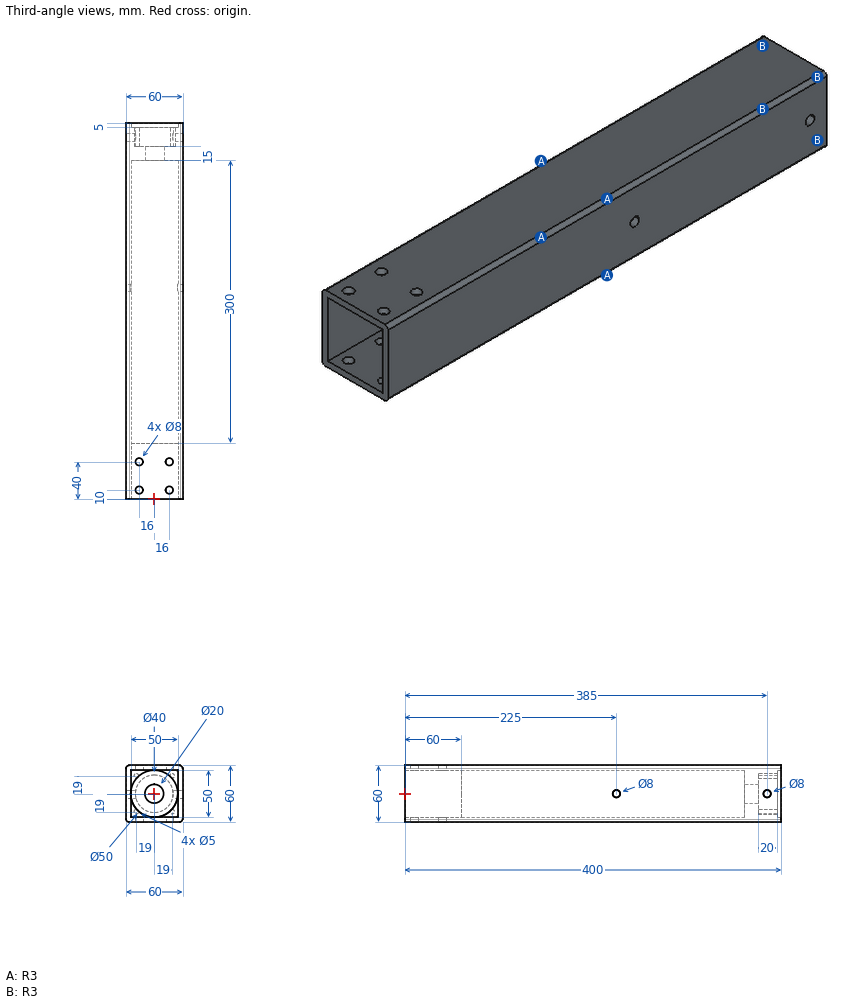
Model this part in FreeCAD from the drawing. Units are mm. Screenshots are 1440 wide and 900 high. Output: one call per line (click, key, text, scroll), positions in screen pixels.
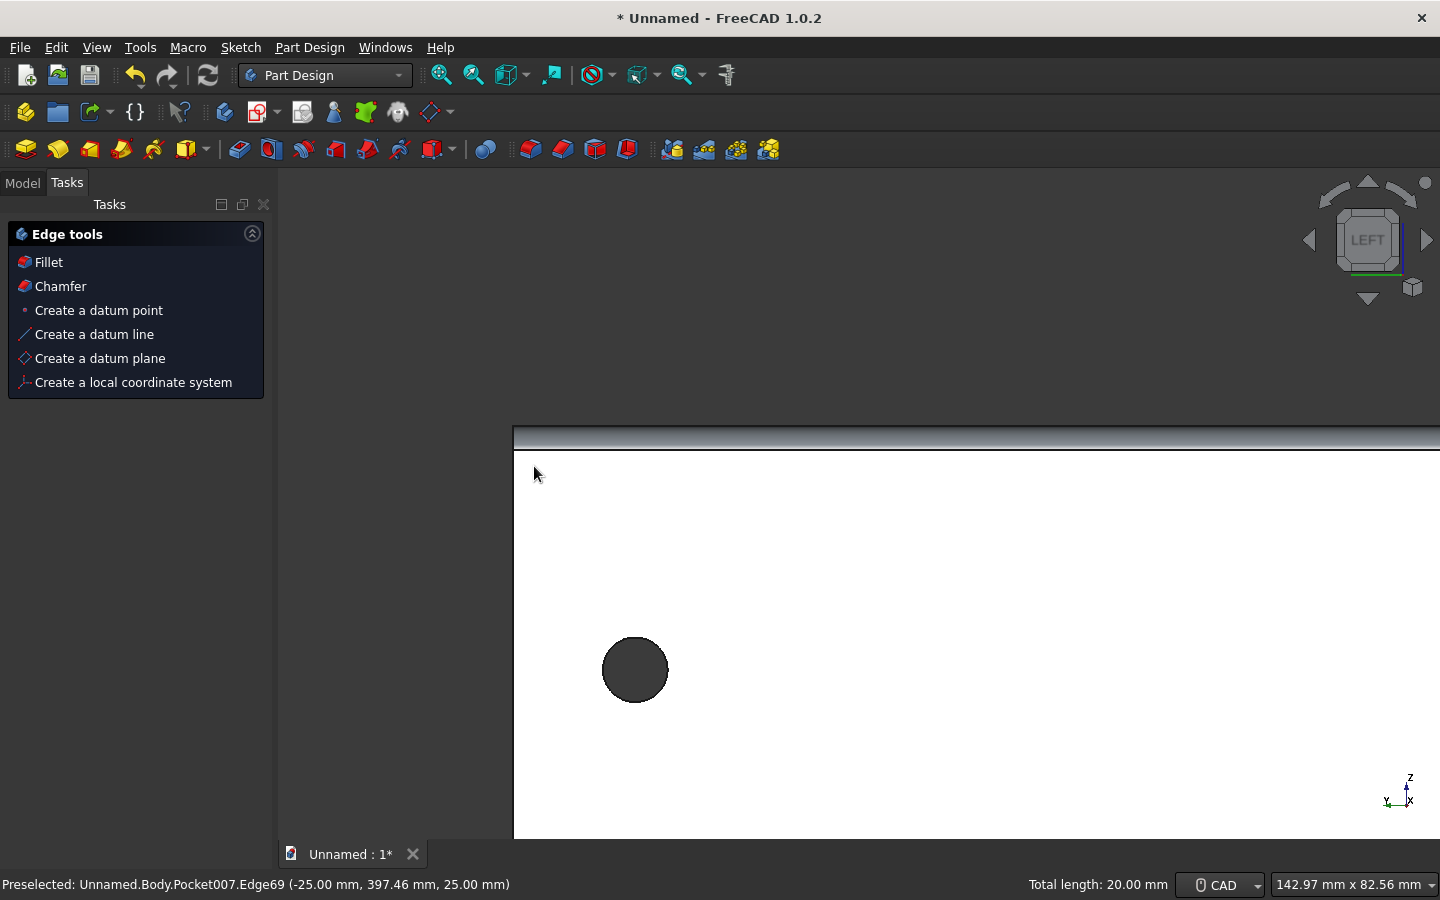
click(532, 150)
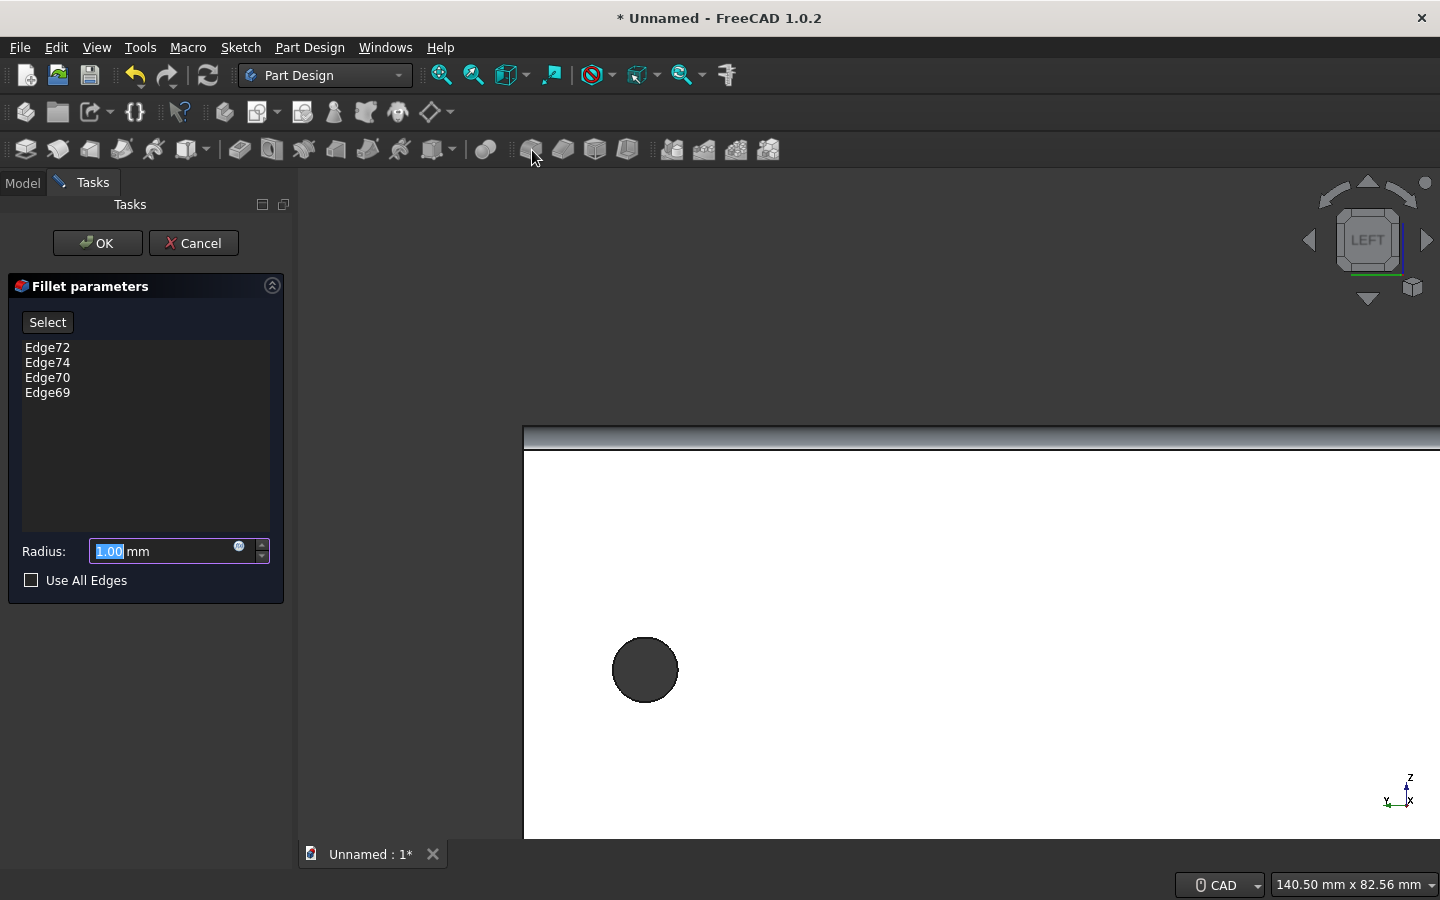
text(3)
key(Tab)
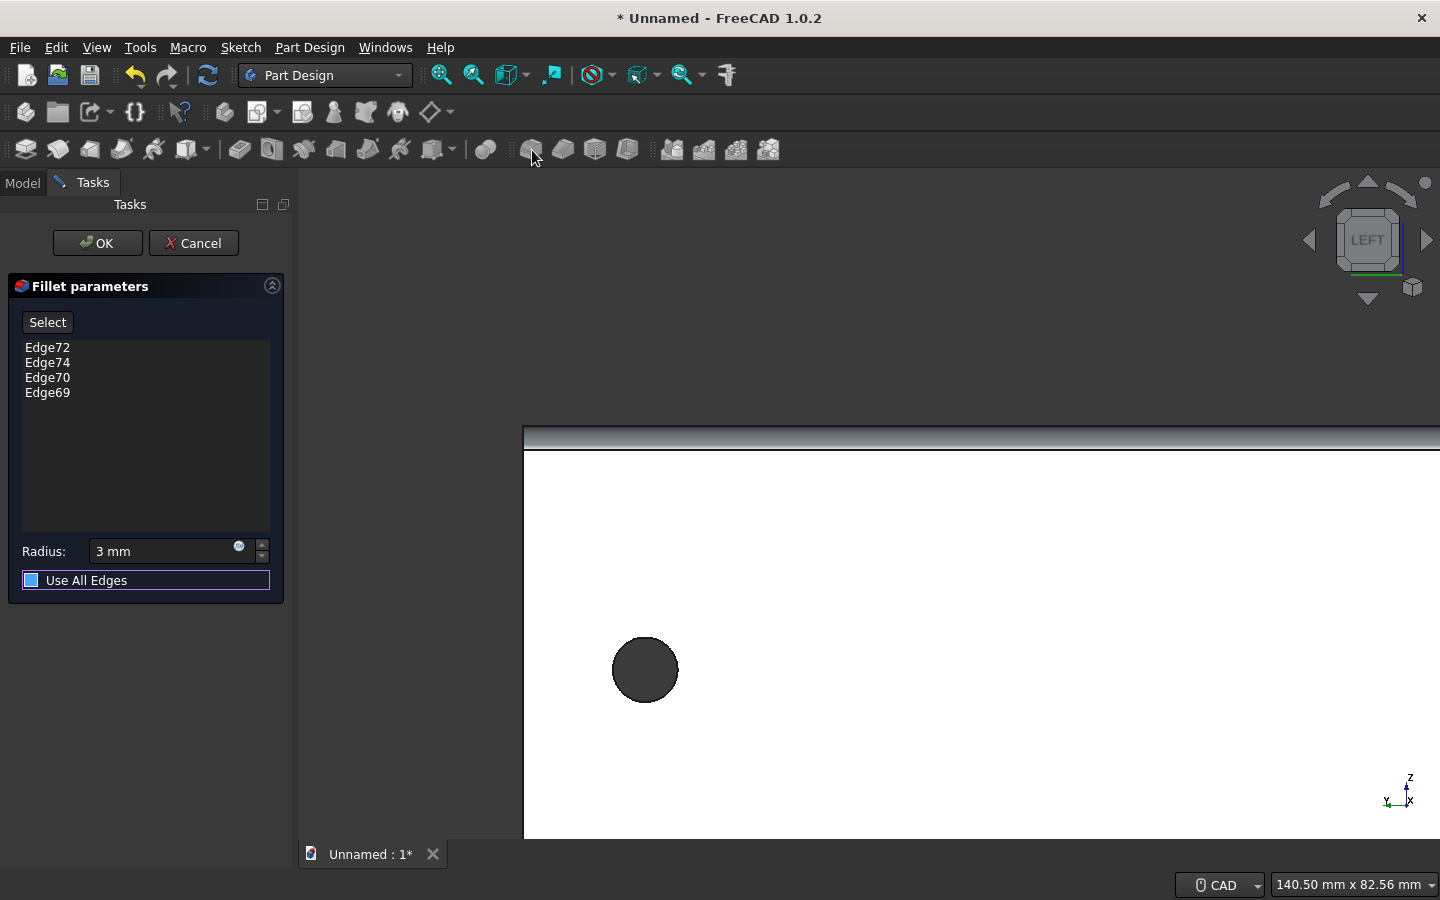
click(98, 243)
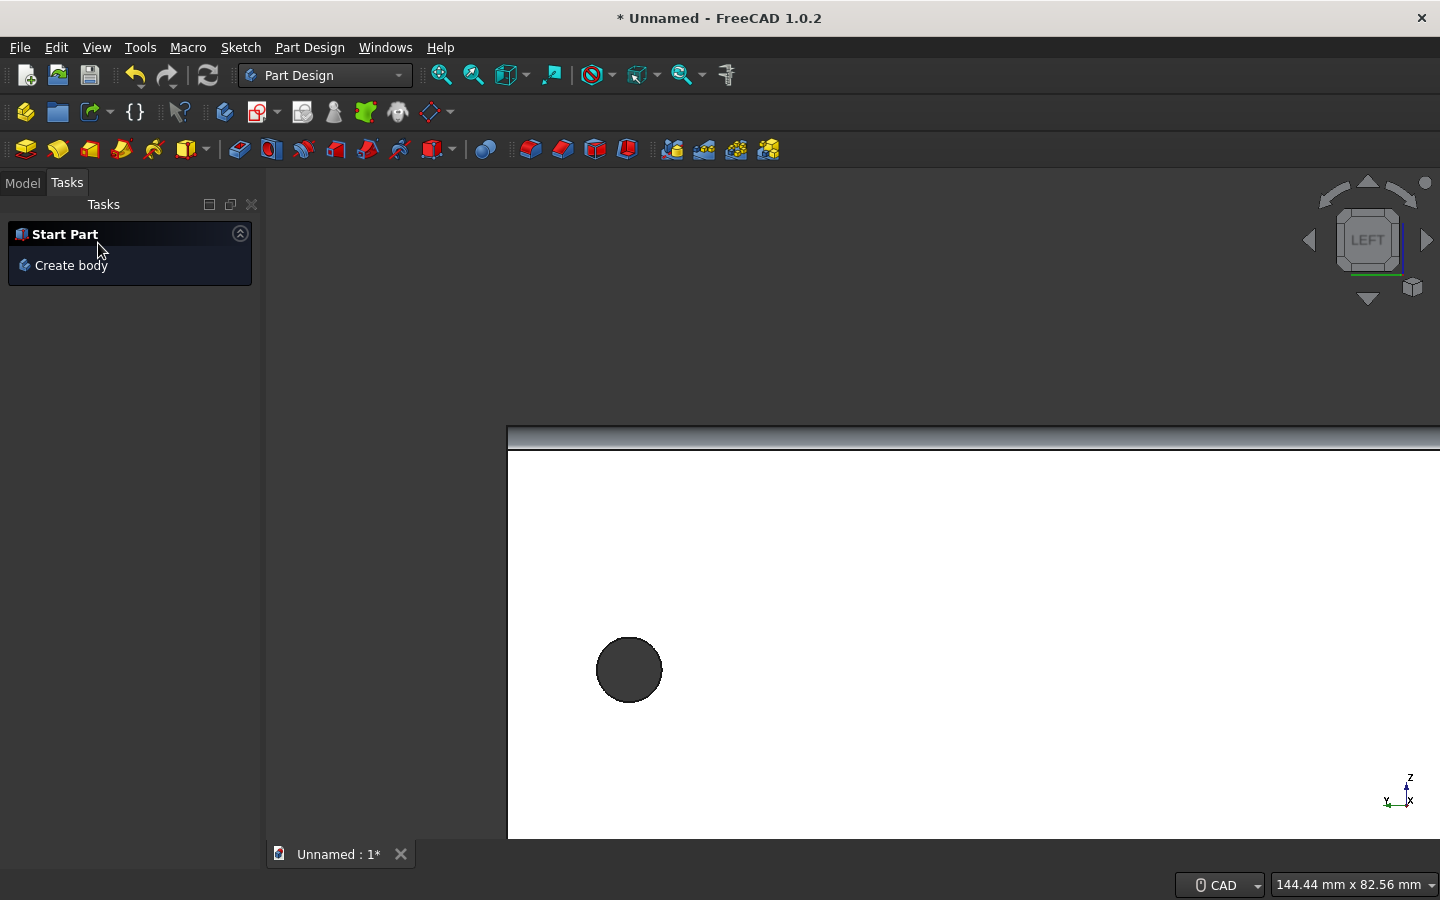
click(442, 76)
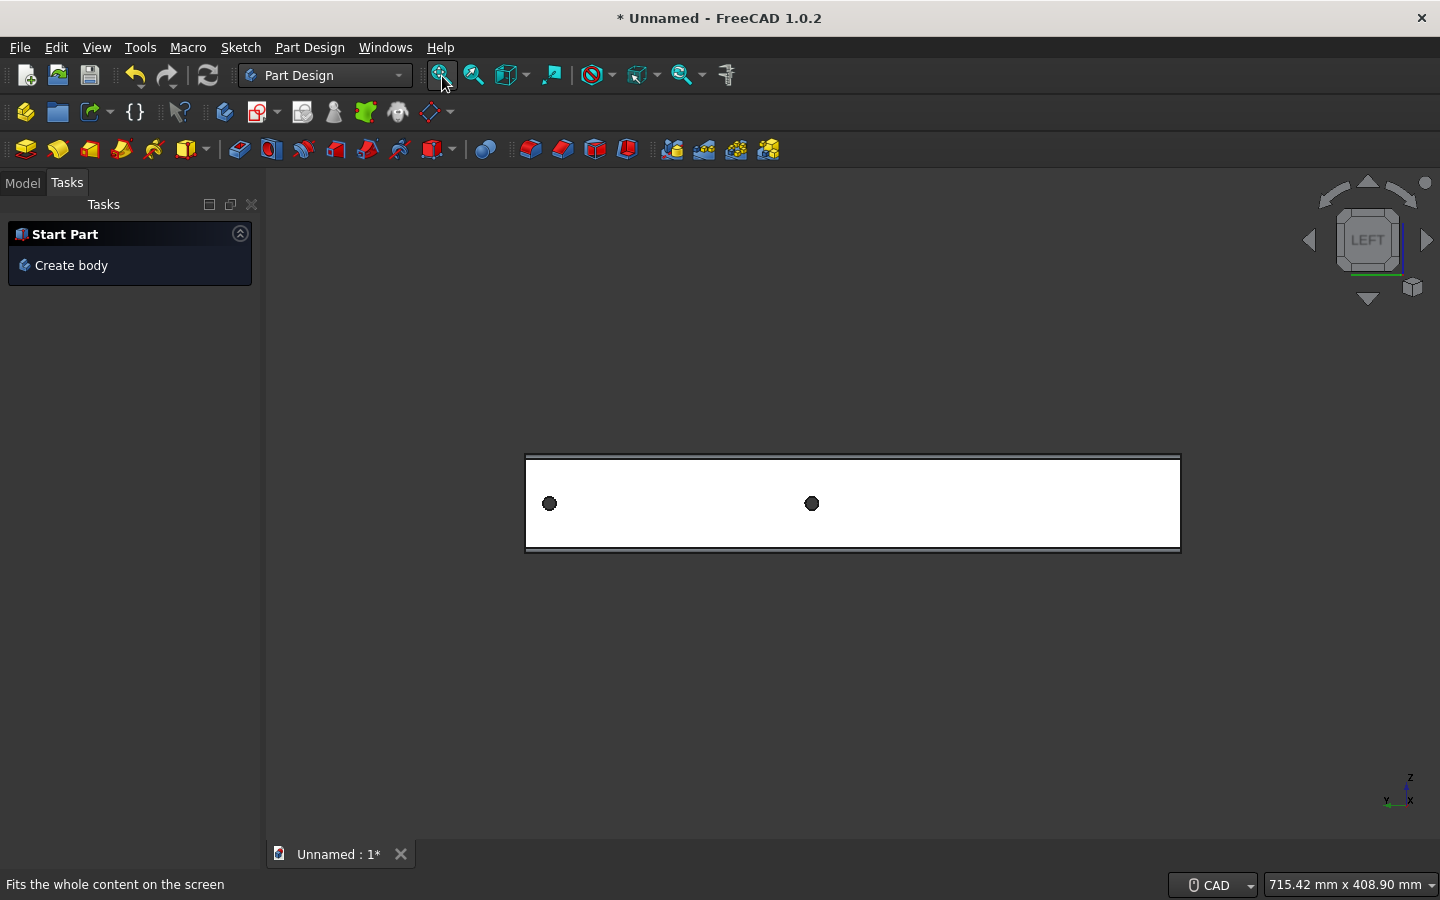
key(4)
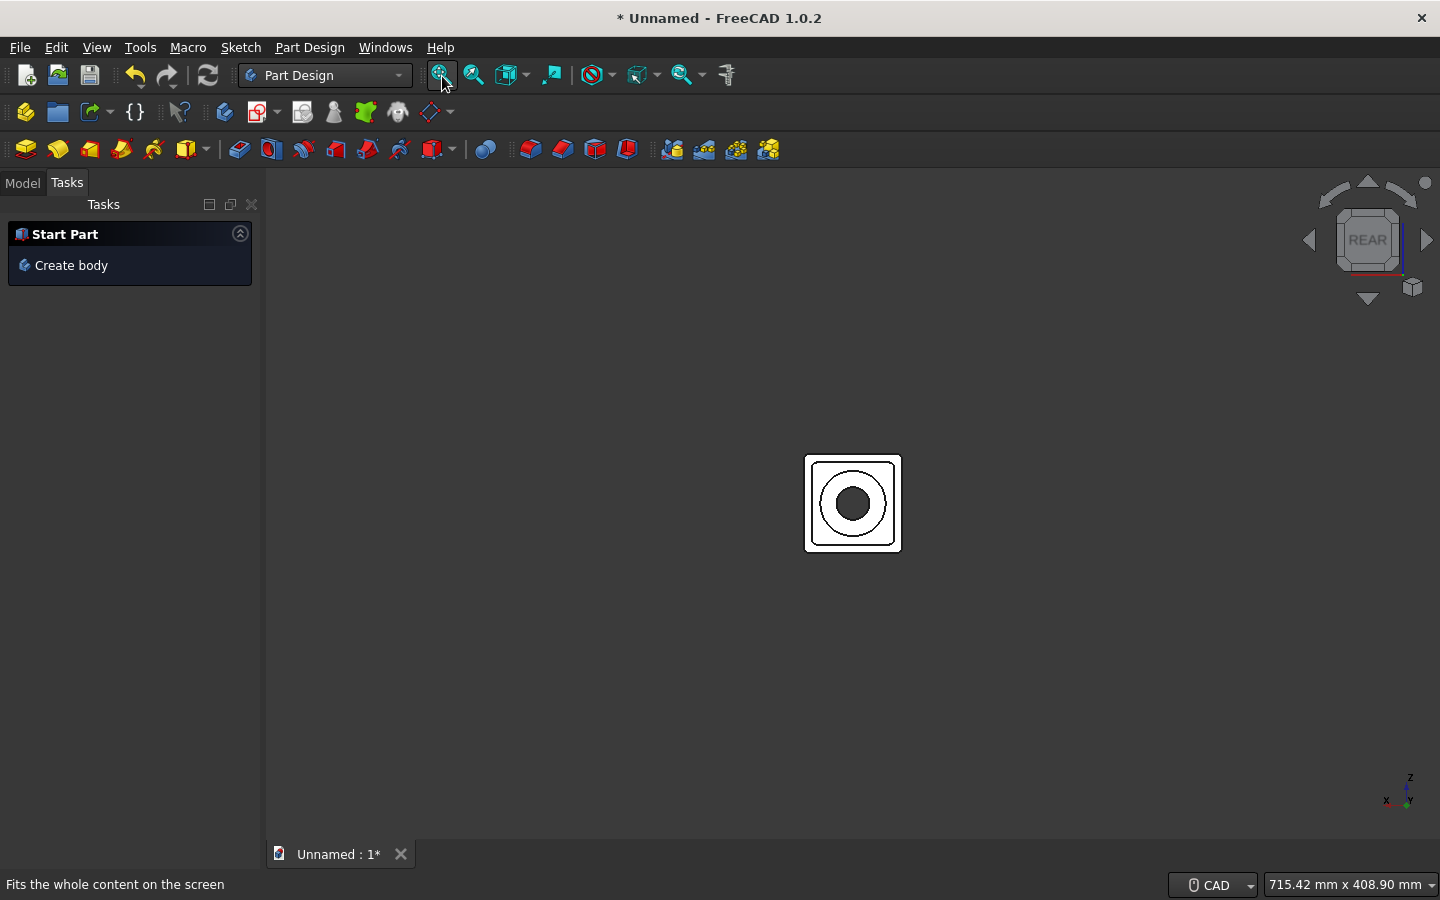
click(442, 76)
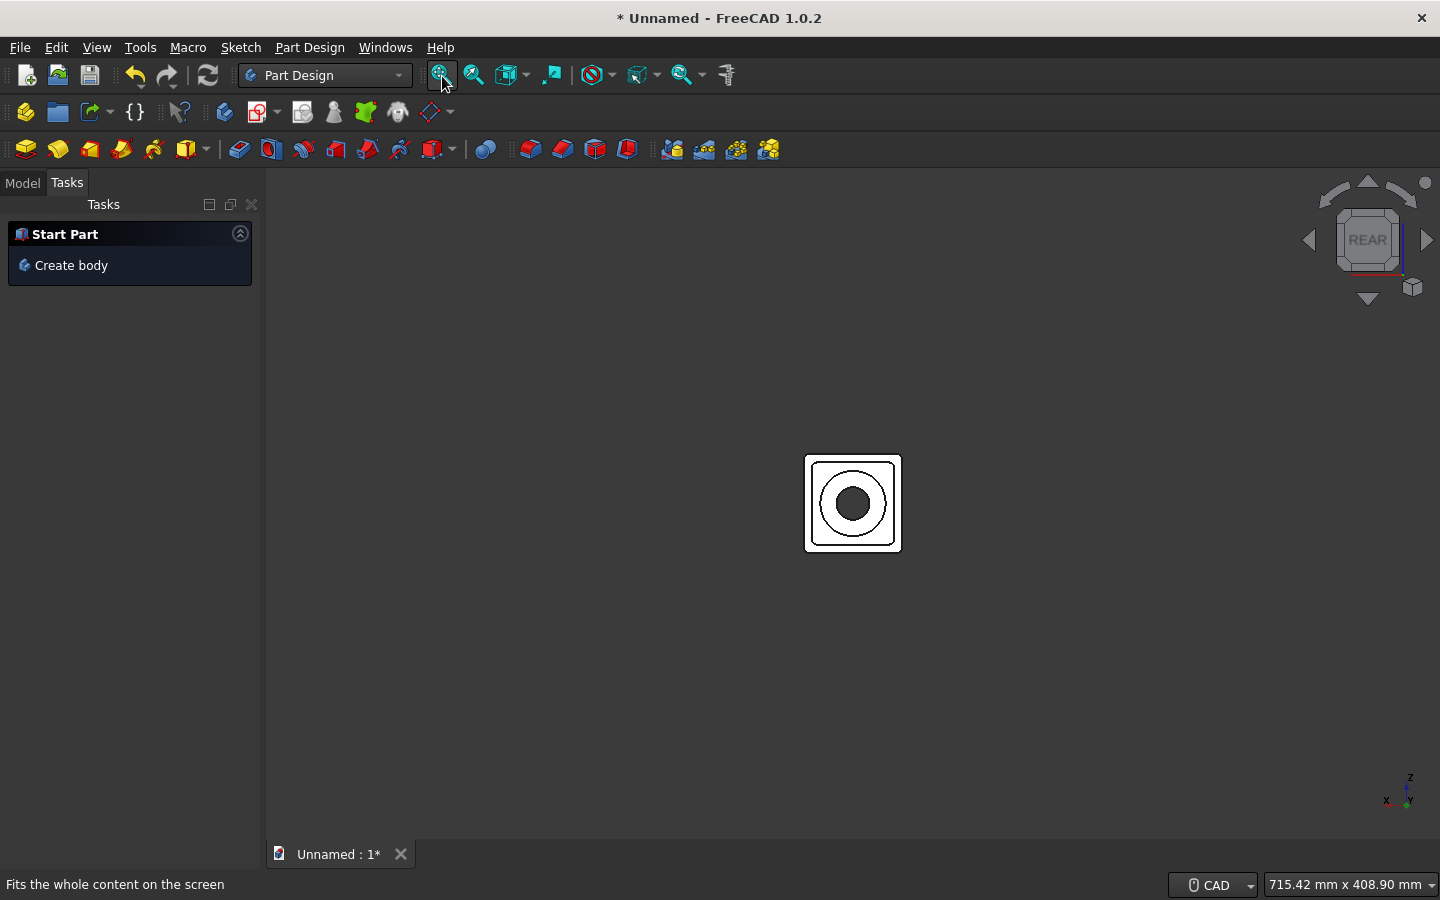
scroll(818, 467, up, 4)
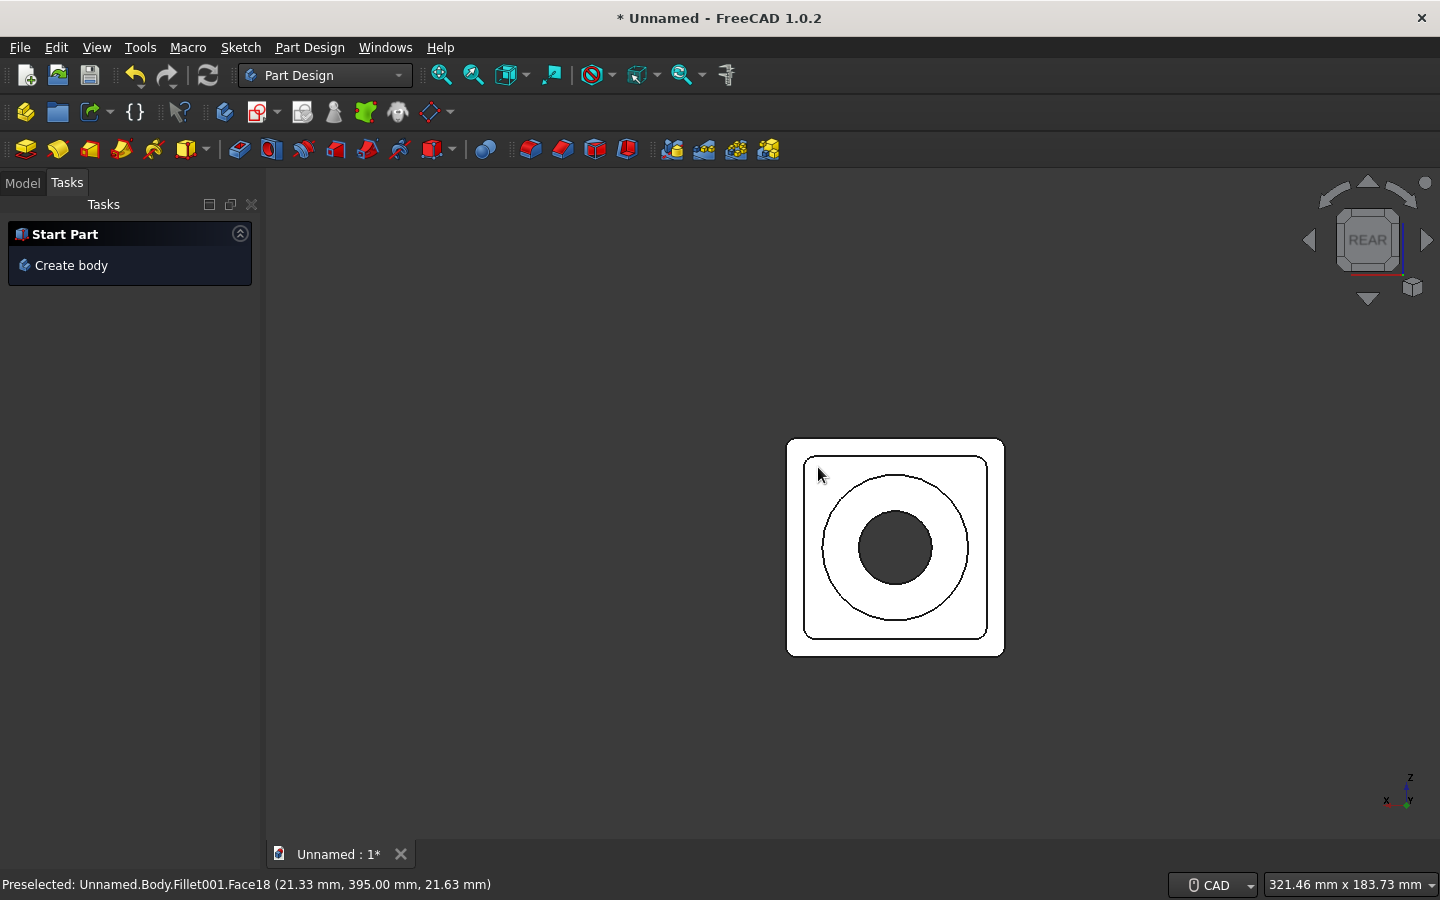
click(817, 468)